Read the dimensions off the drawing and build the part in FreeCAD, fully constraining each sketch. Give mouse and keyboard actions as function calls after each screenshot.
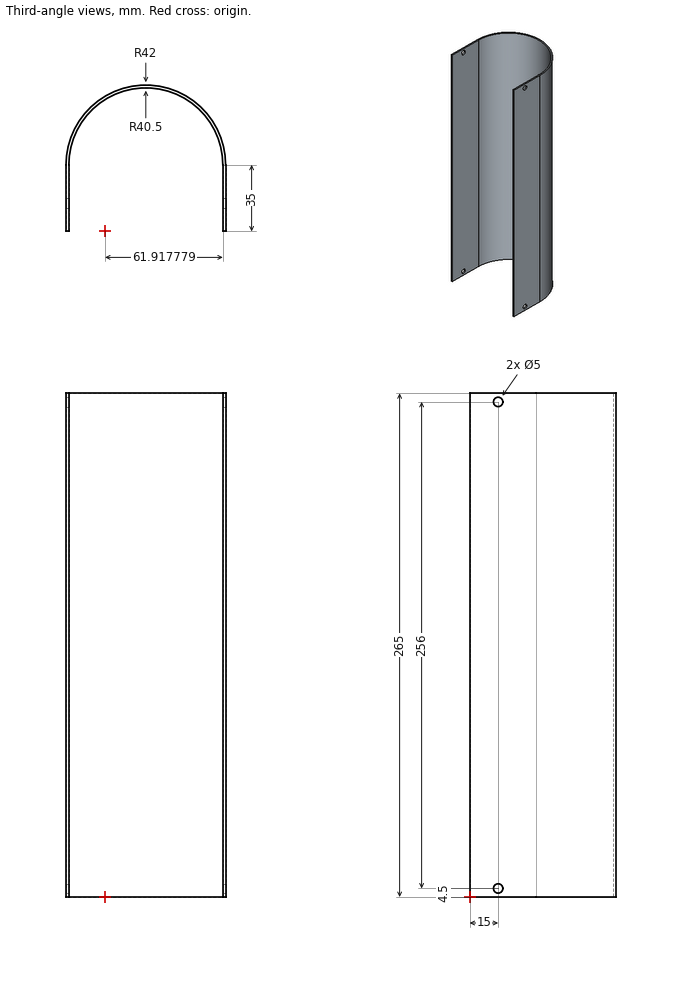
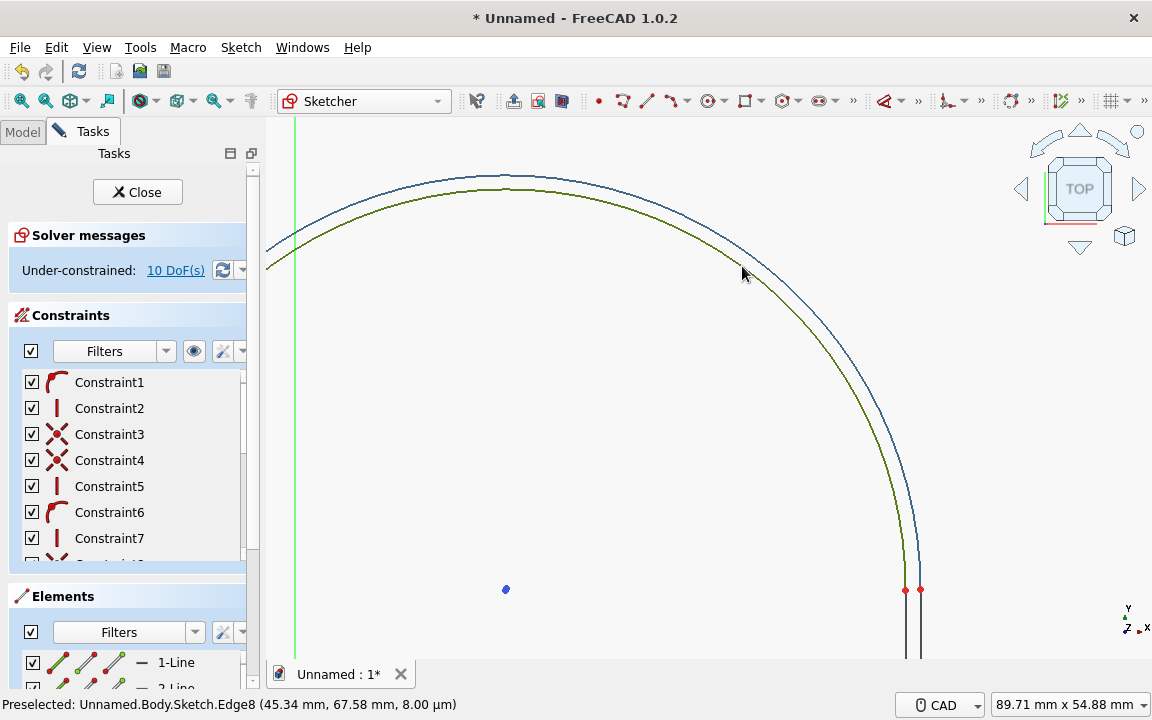
key(c)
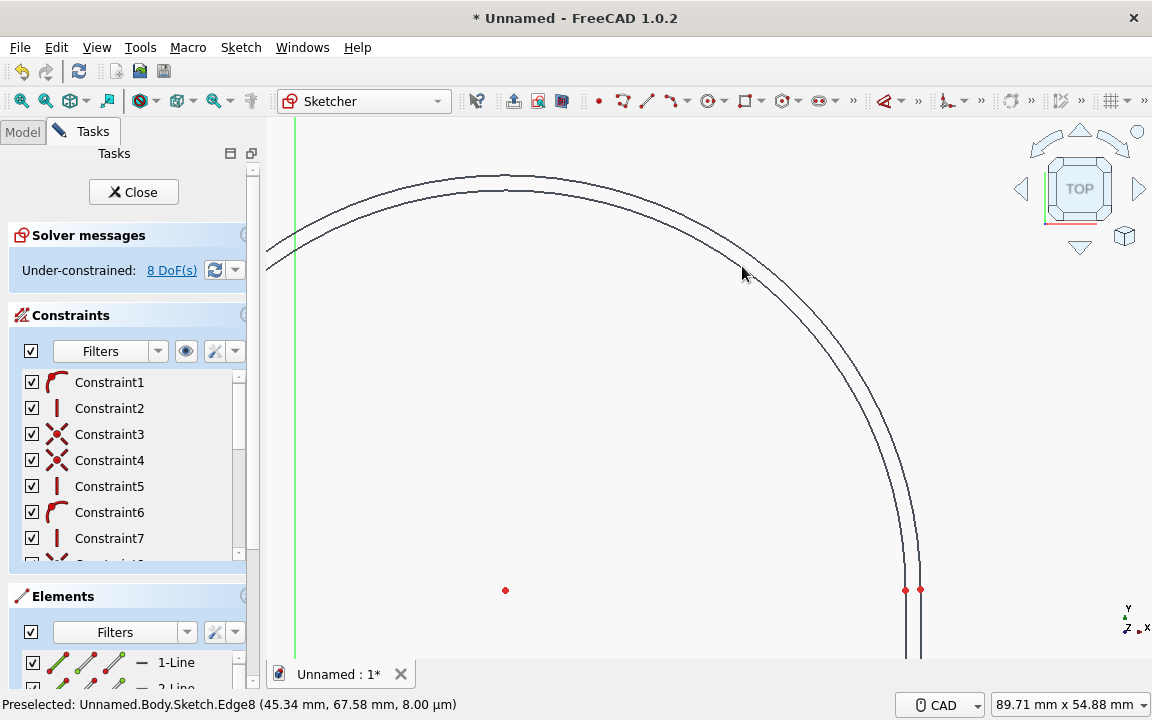
click(749, 254)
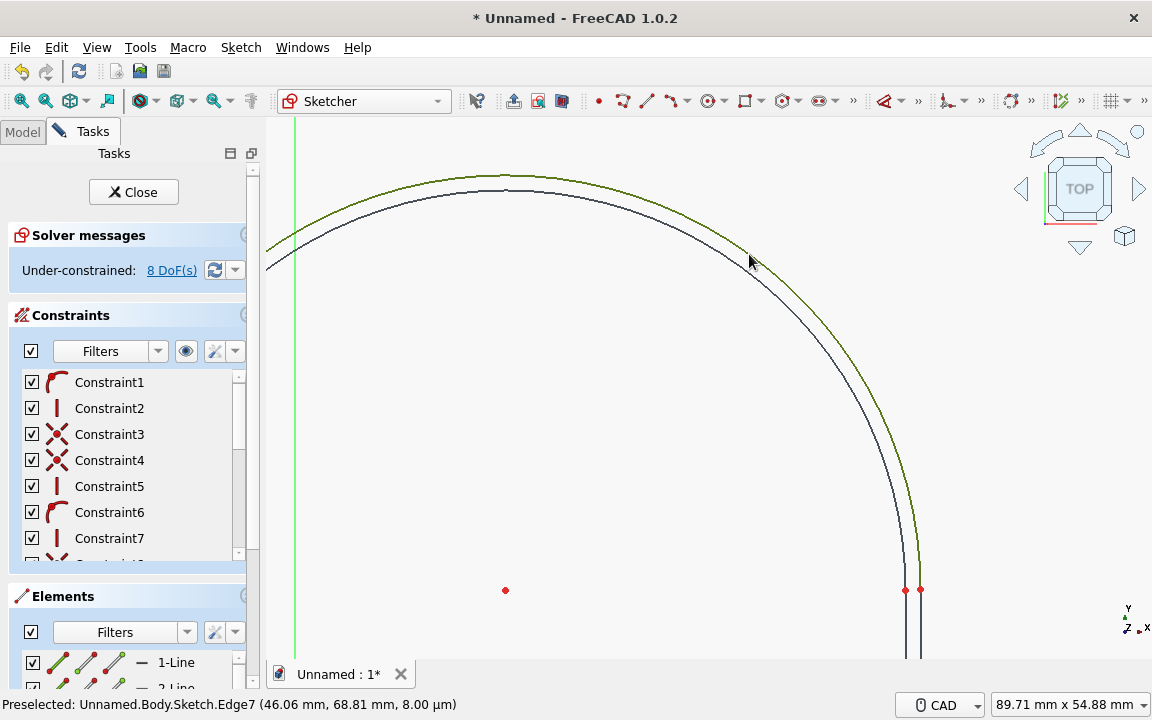
key(k)
key(r)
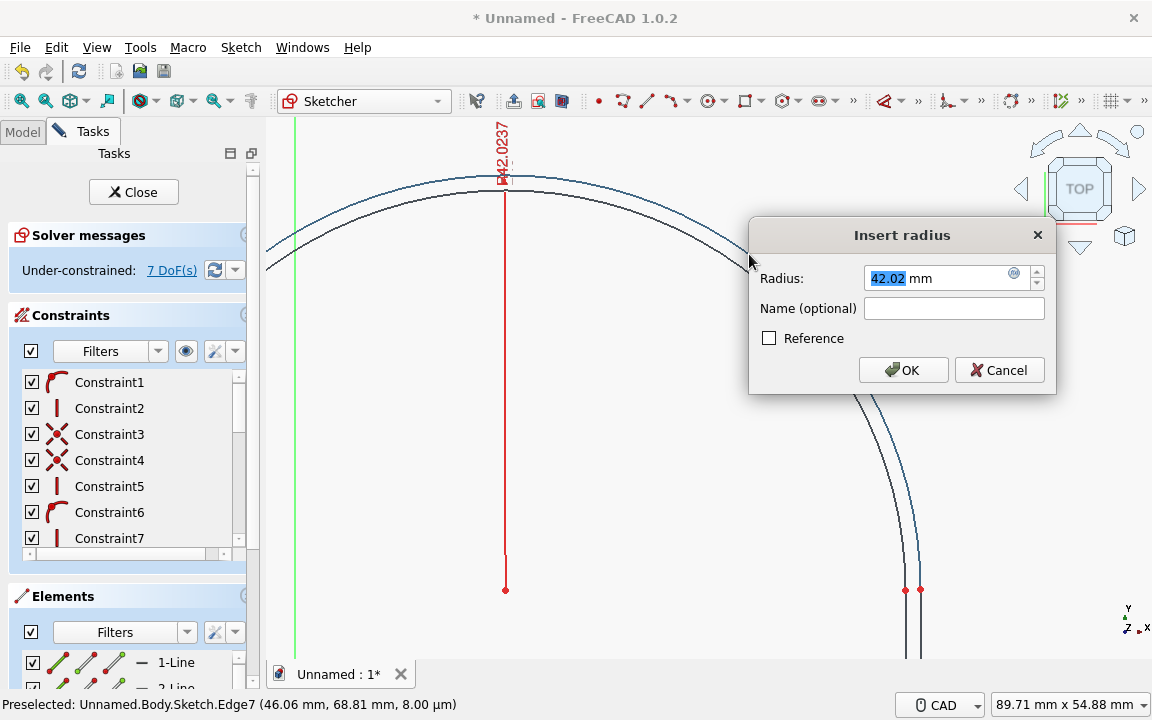
text(42)
key(Return)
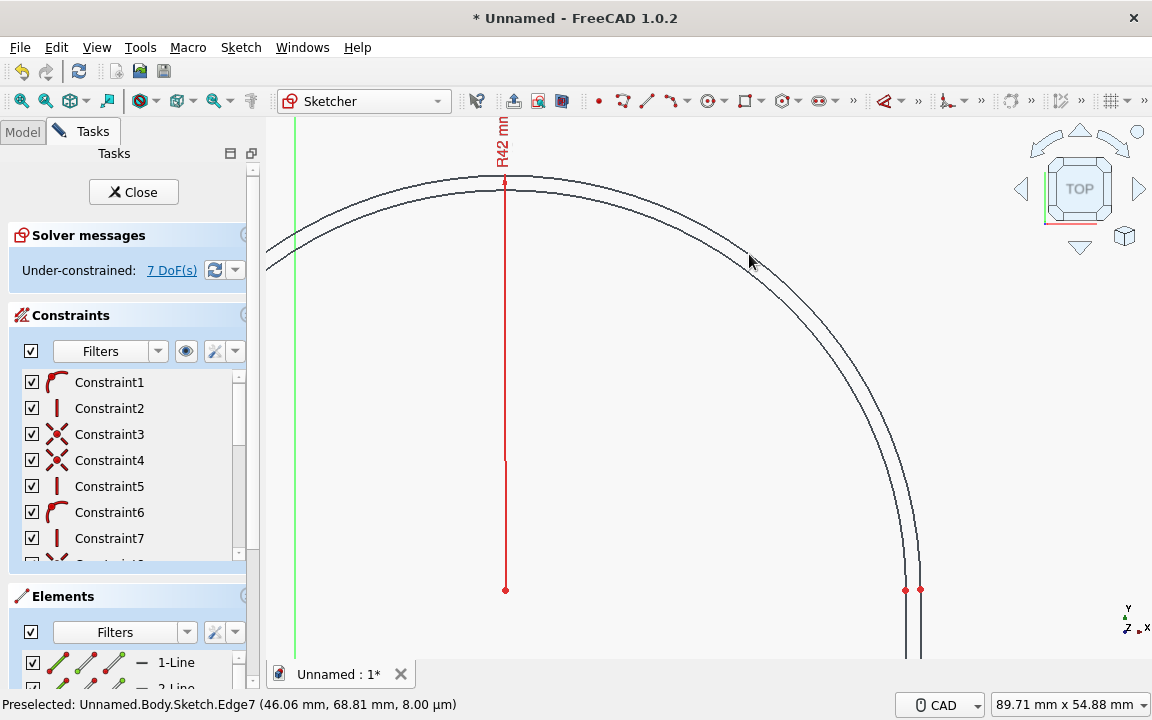
click(741, 267)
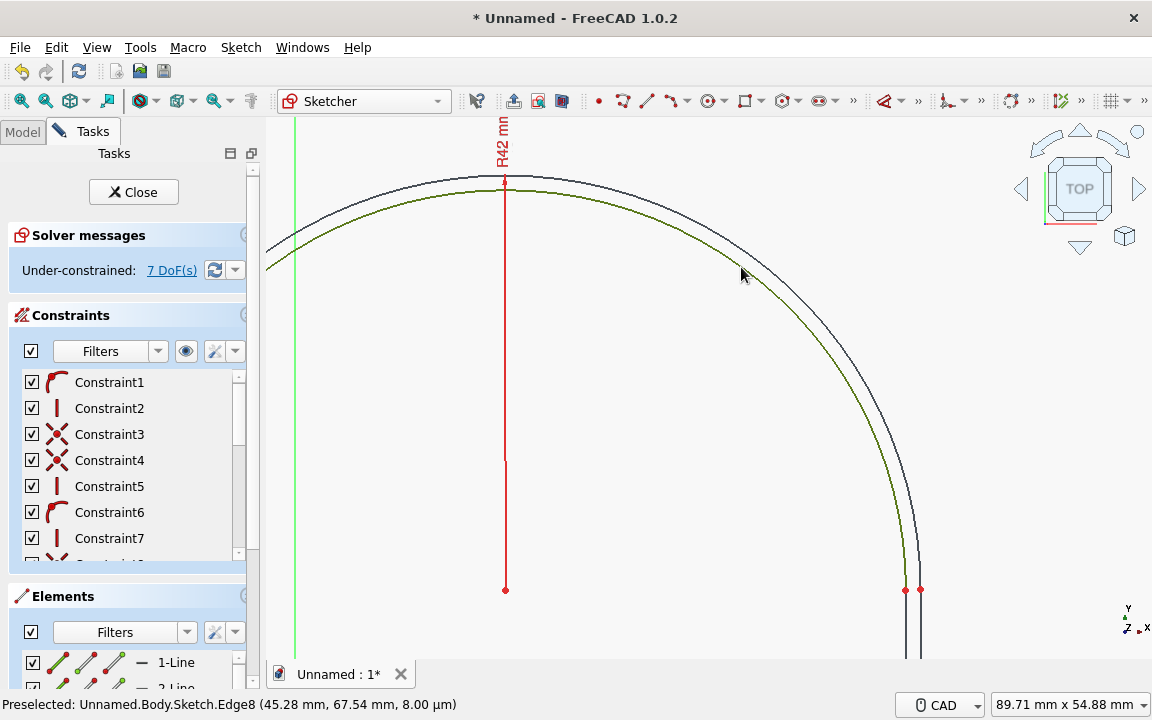
key(k)
key(r)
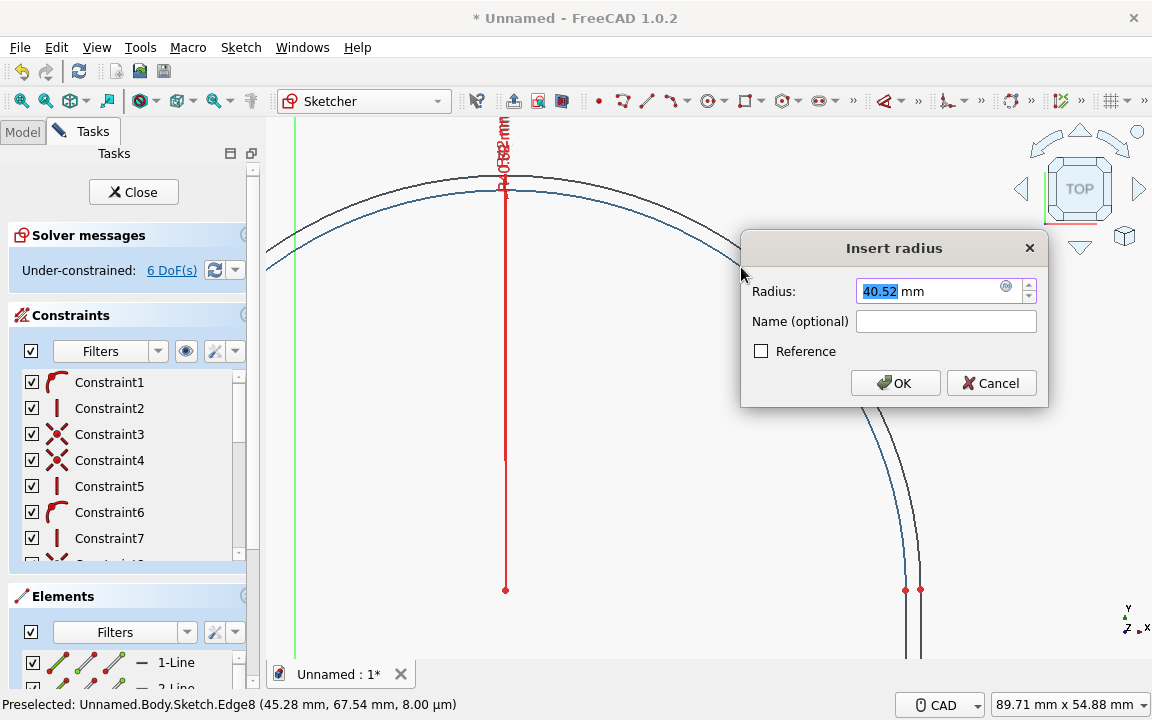
text(40.5)
key(Return)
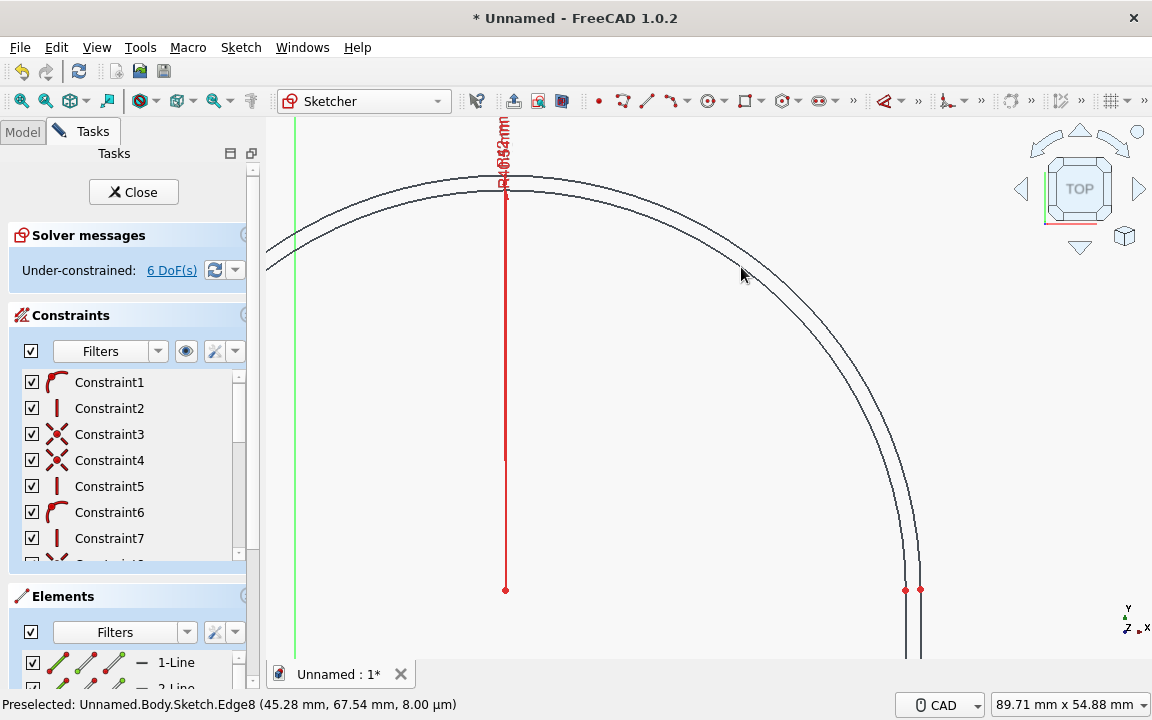
scroll(750, 253, down, 4)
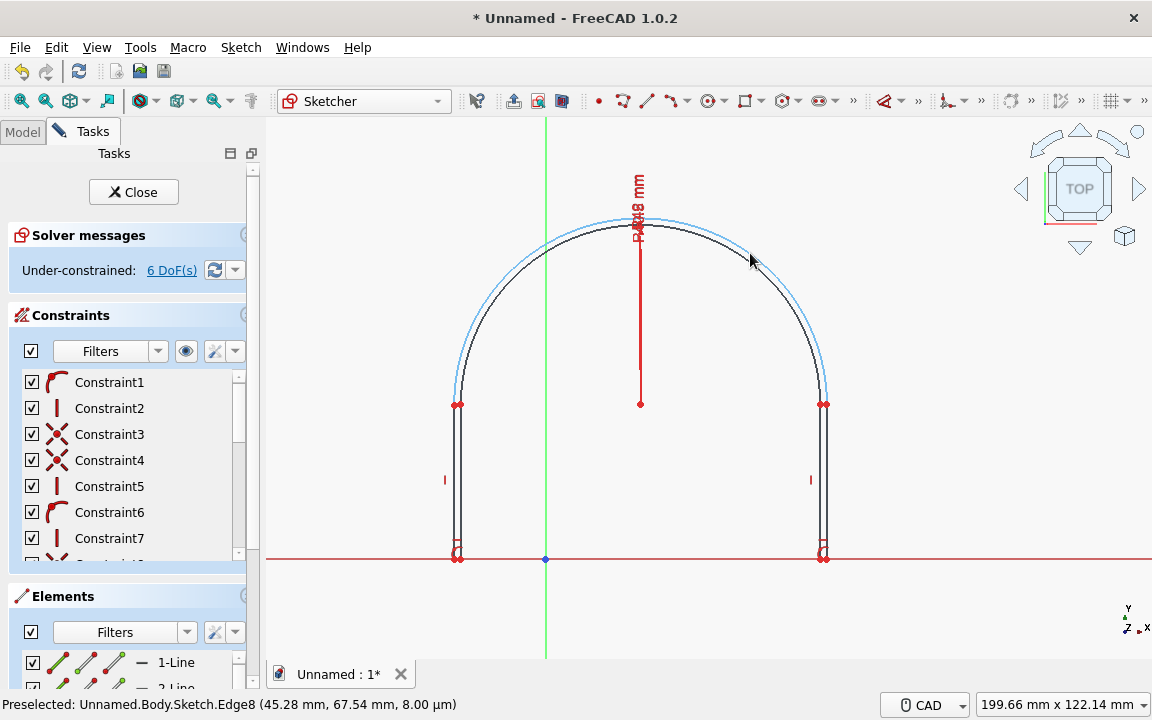
scroll(820, 451, up, 4)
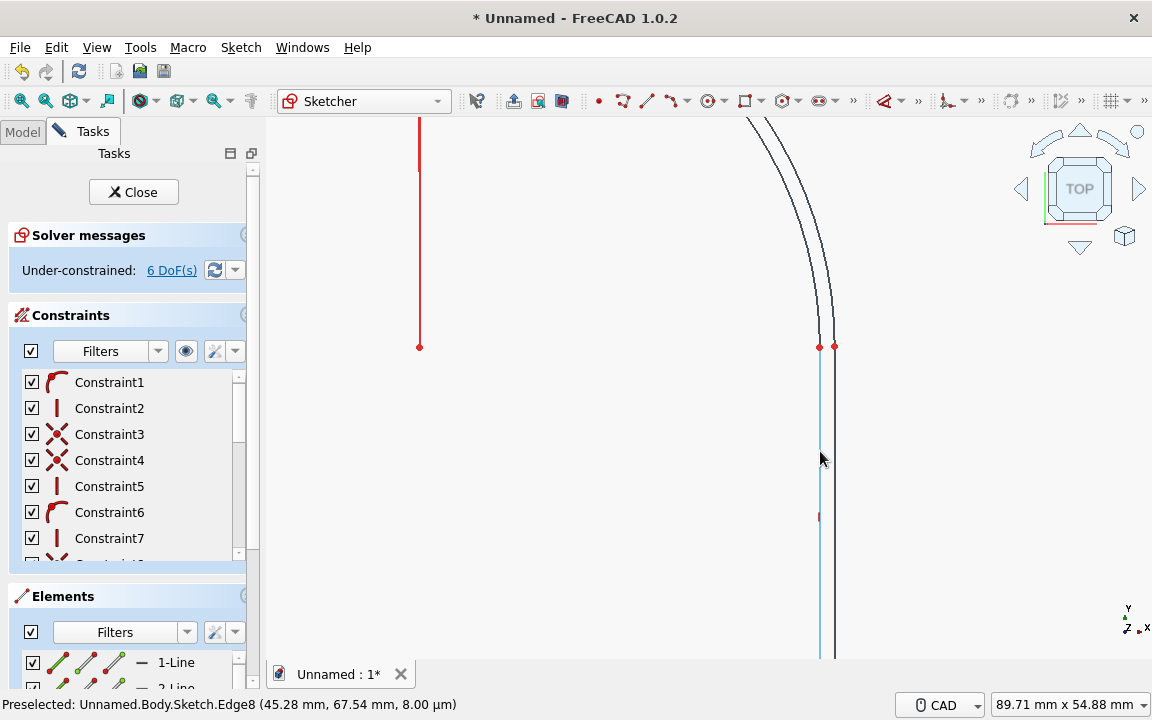
click(820, 450)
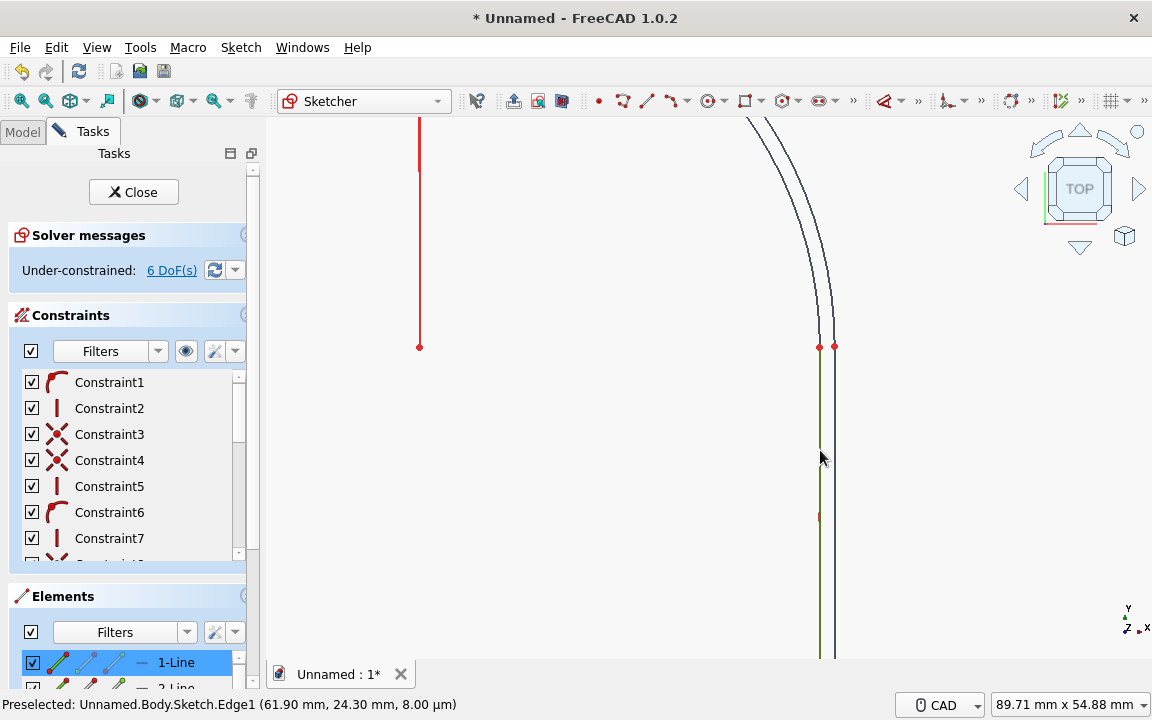
key(i)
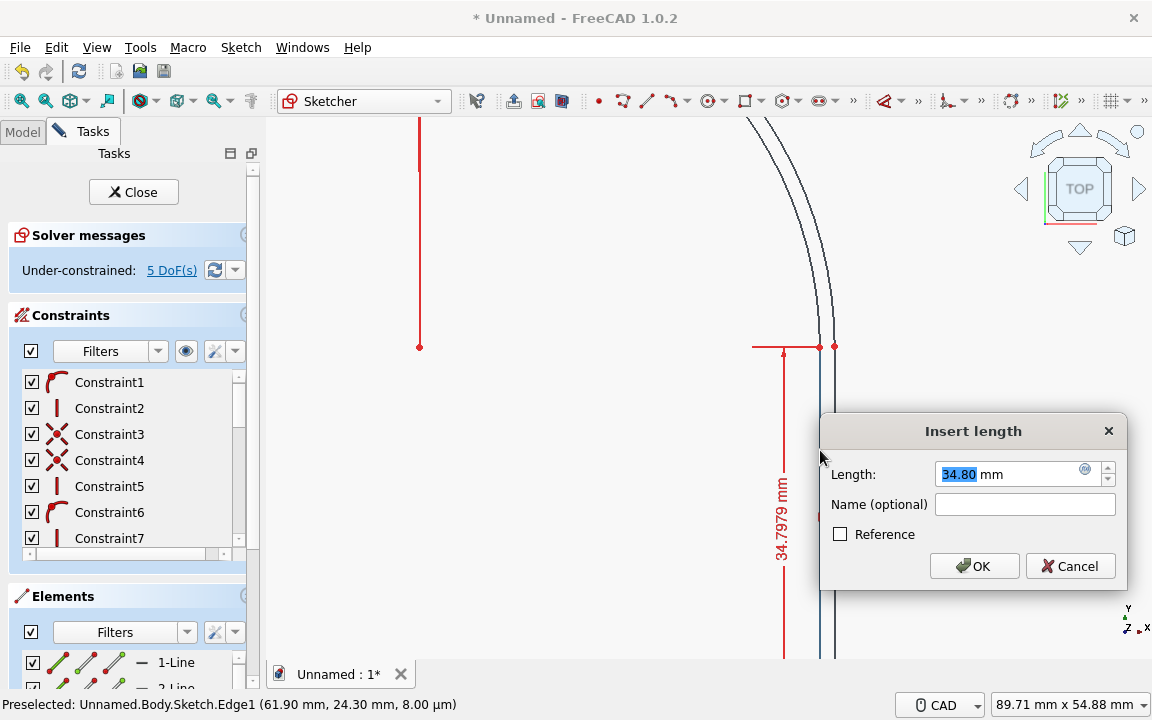
text(35)
key(Return)